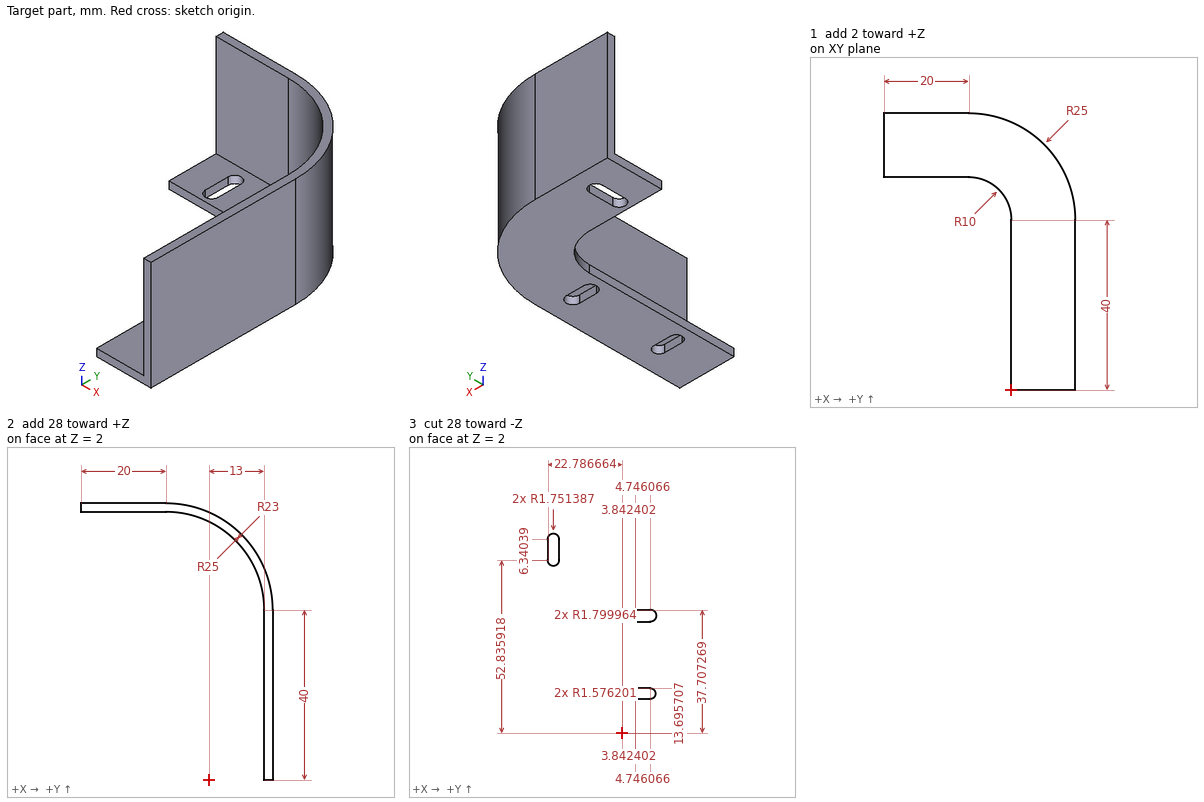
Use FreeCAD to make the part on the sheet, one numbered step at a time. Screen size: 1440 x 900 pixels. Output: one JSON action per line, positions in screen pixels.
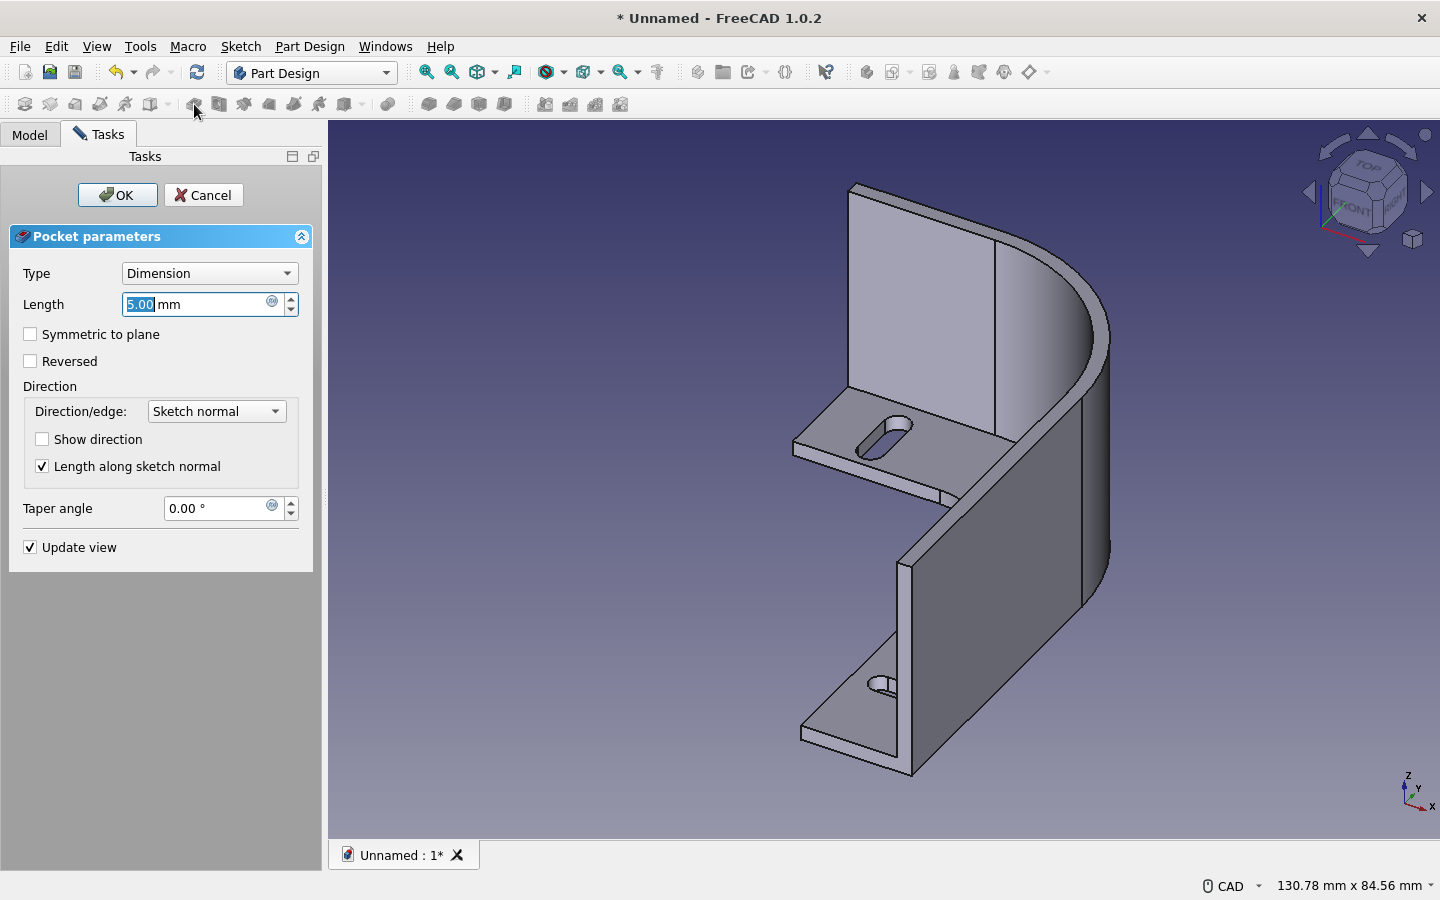
{"action": "type", "text": "28"}
{"action": "key", "text": "Tab"}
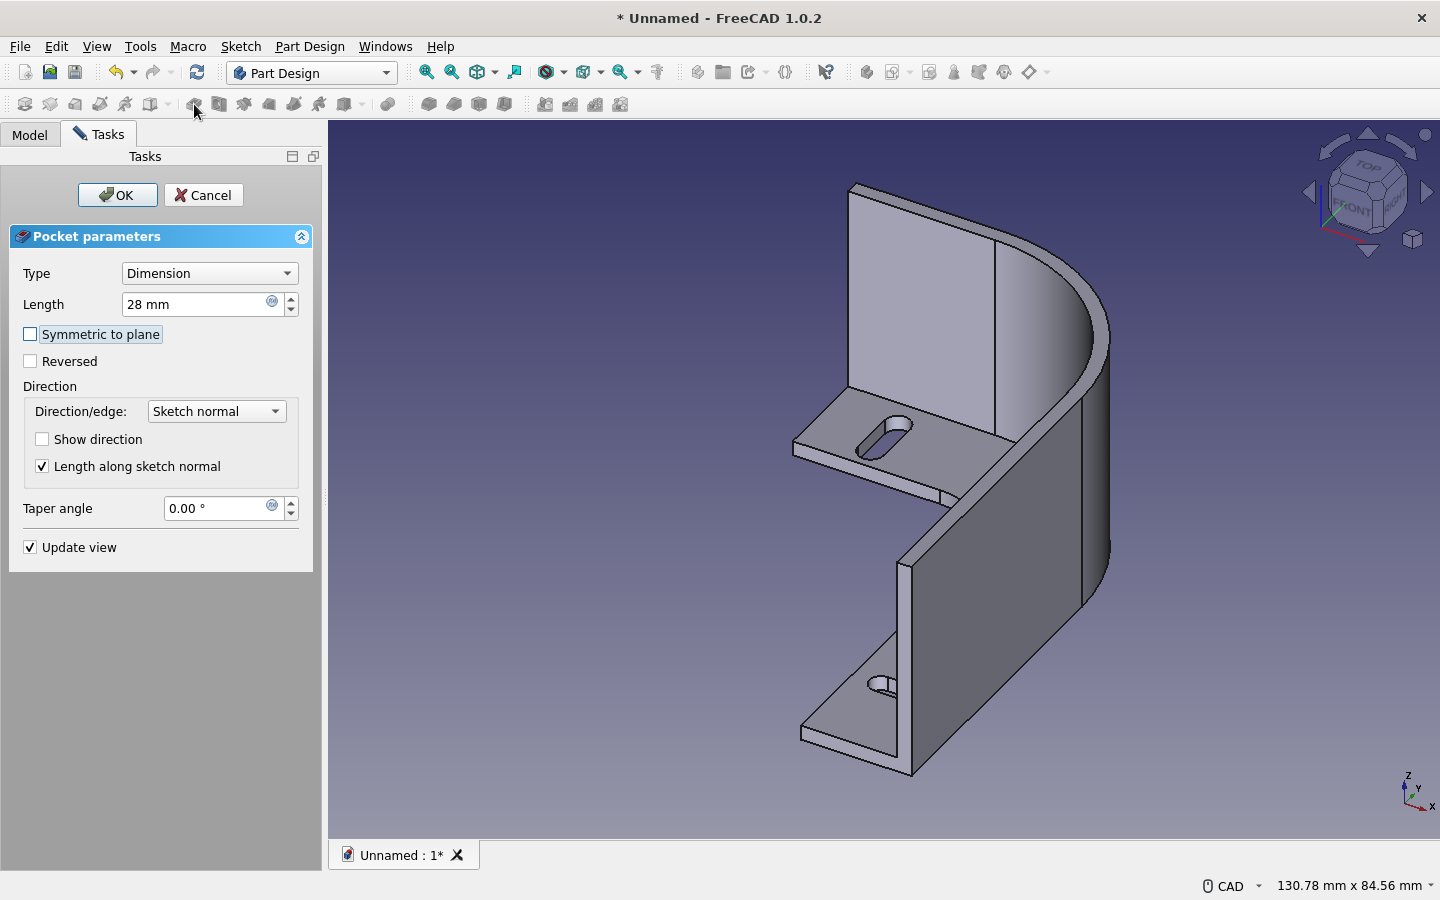
{"action": "left_click", "coordinate": [118, 195]}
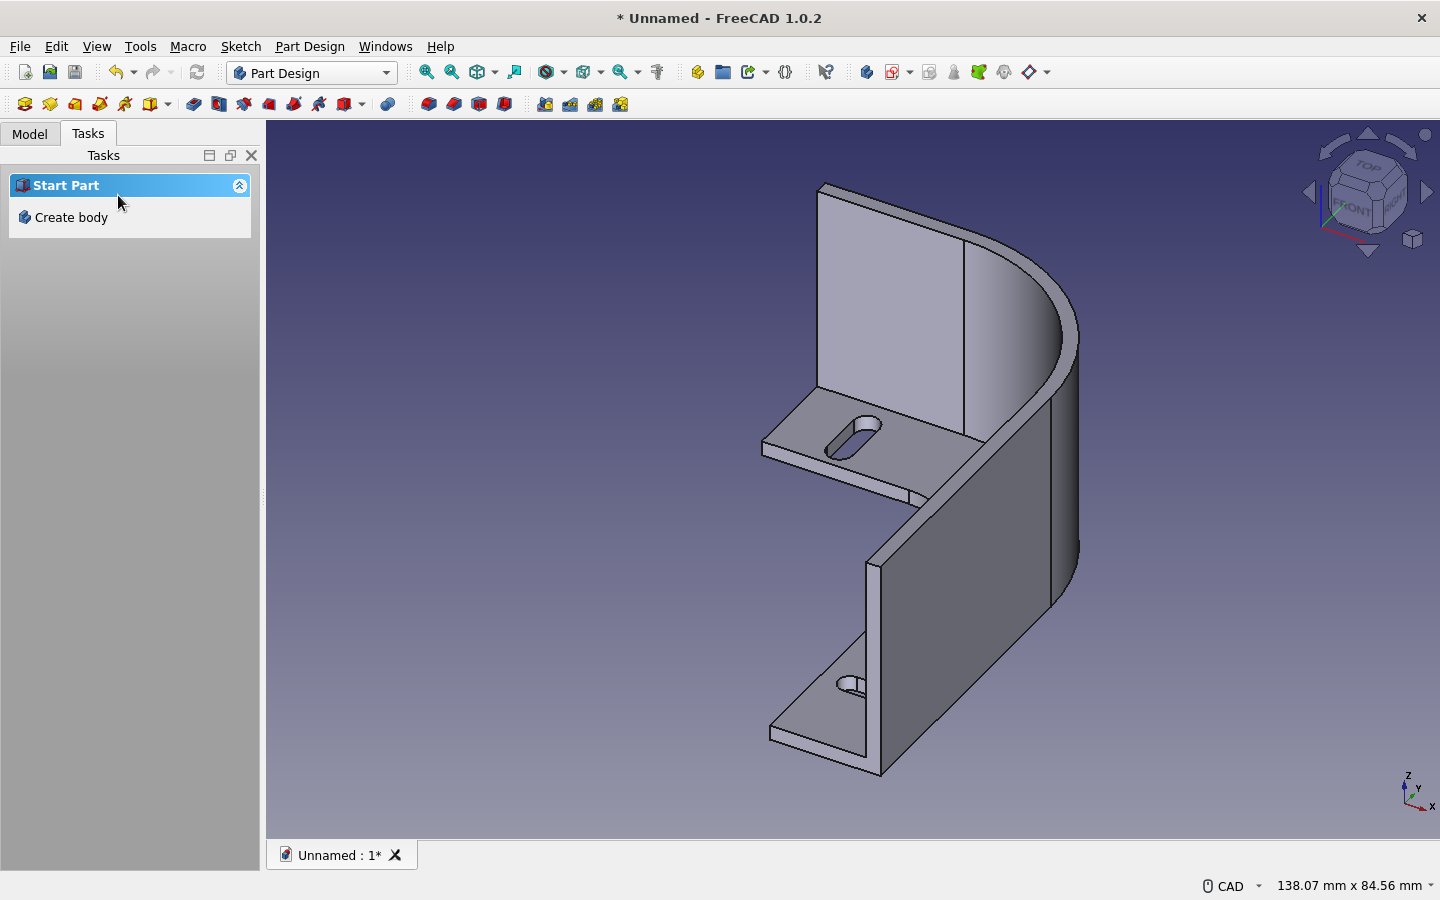
{"action": "key", "text": "0"}